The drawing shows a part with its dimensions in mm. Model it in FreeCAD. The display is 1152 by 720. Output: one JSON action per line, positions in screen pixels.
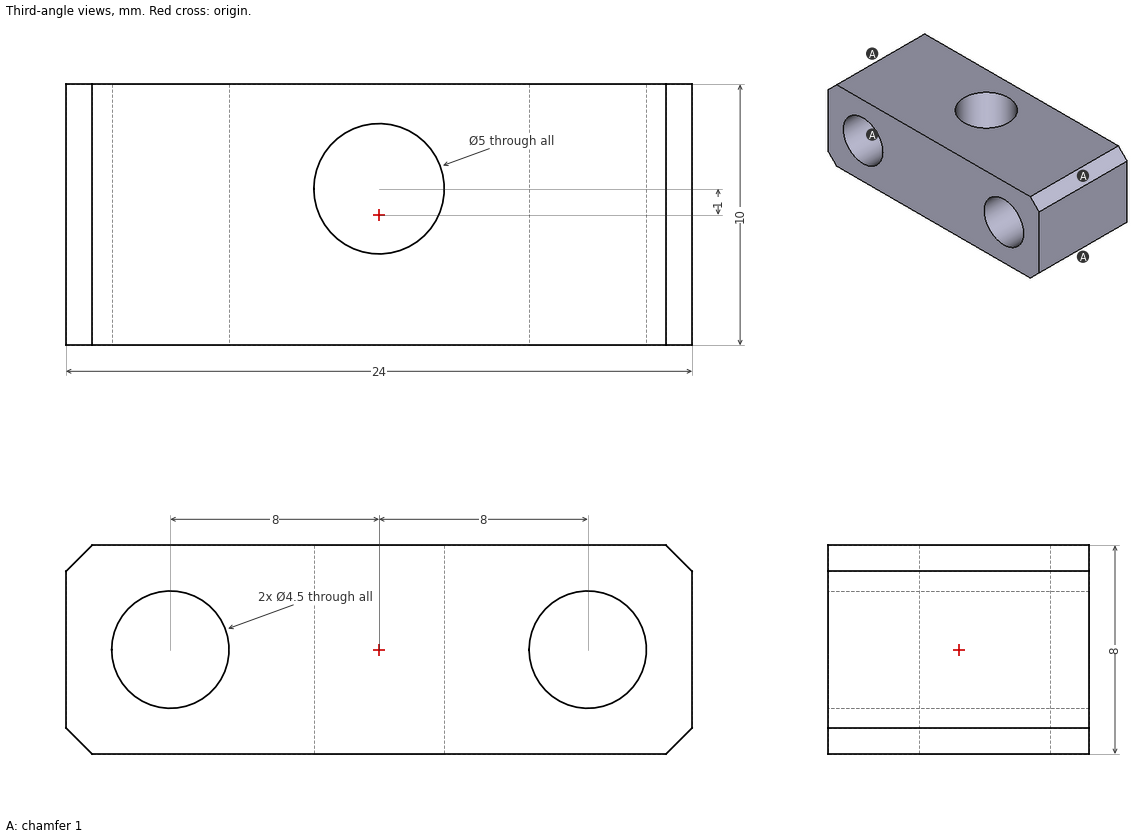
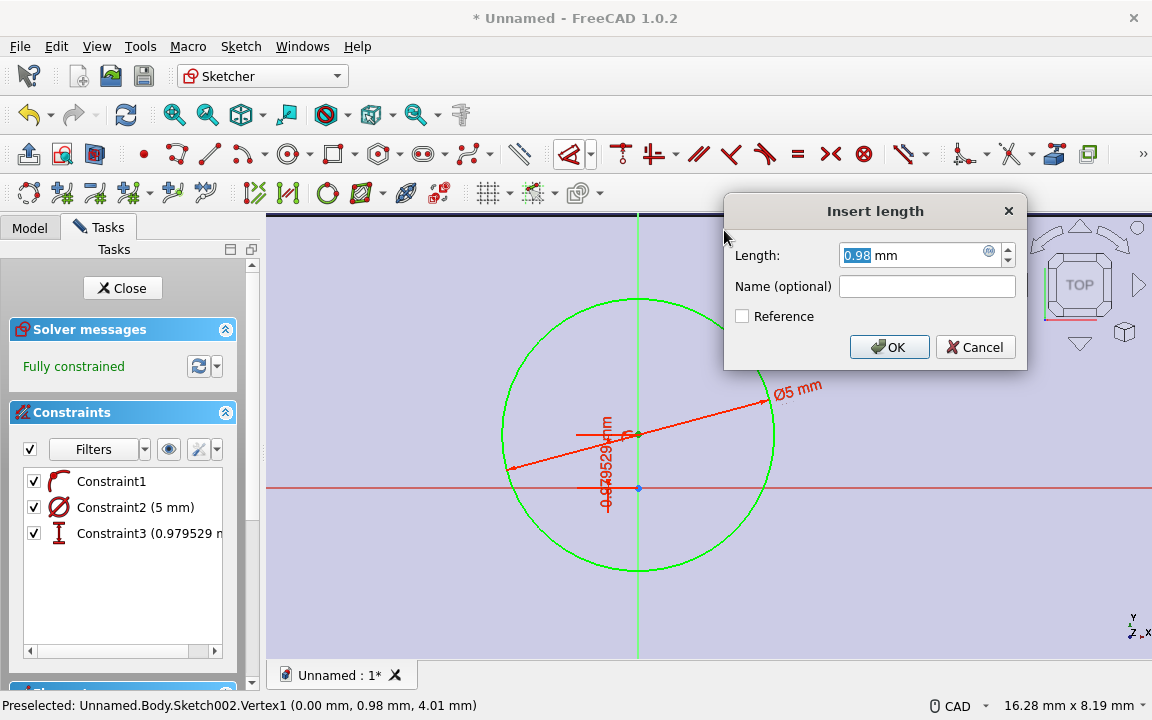
{"action": "type", "text": "1"}
{"action": "key", "text": "Return"}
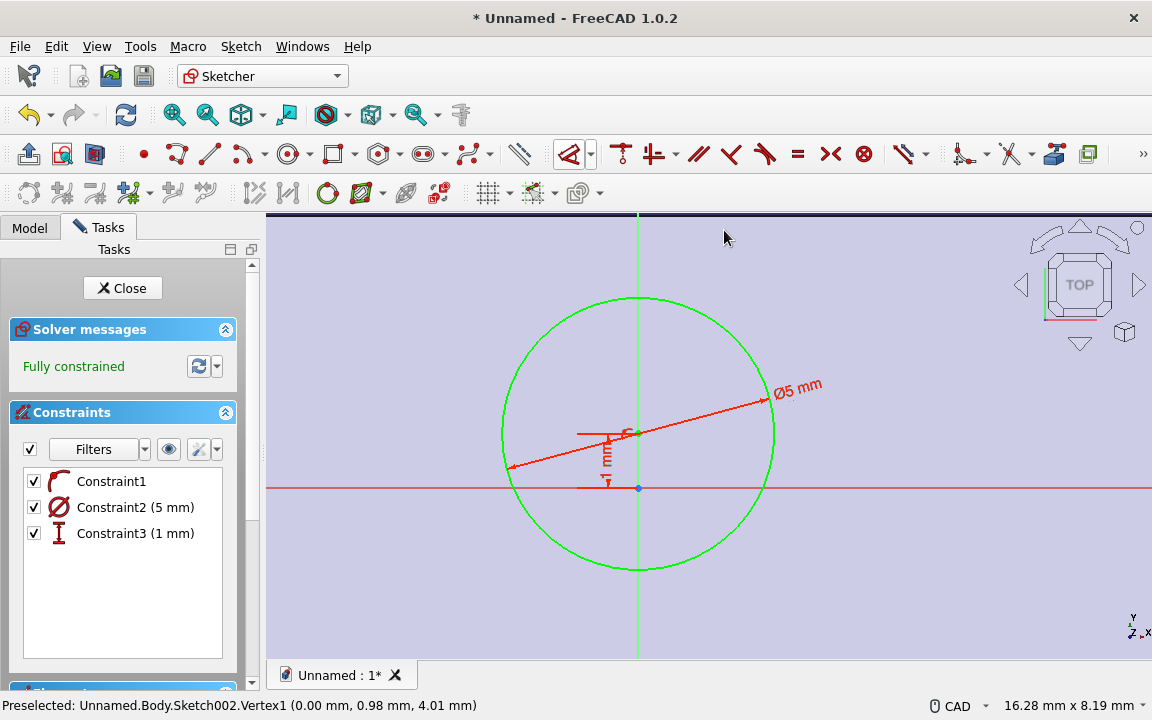
{"action": "left_click", "coordinate": [123, 288]}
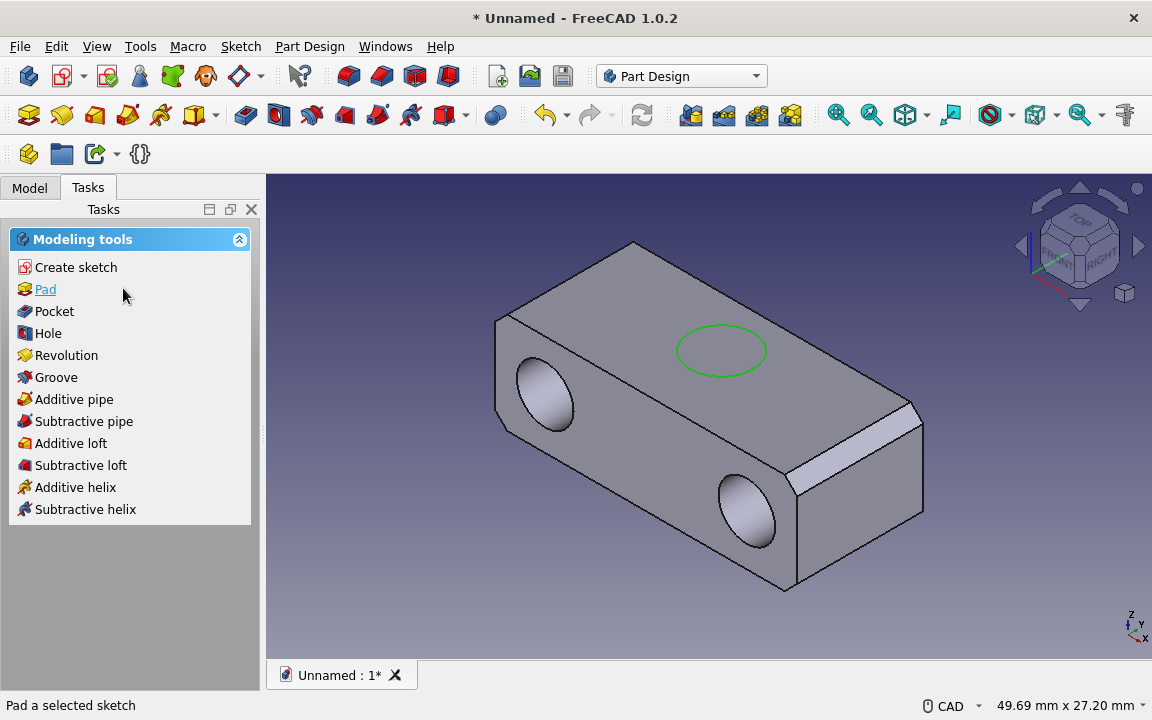
{"action": "left_click", "coordinate": [279, 116]}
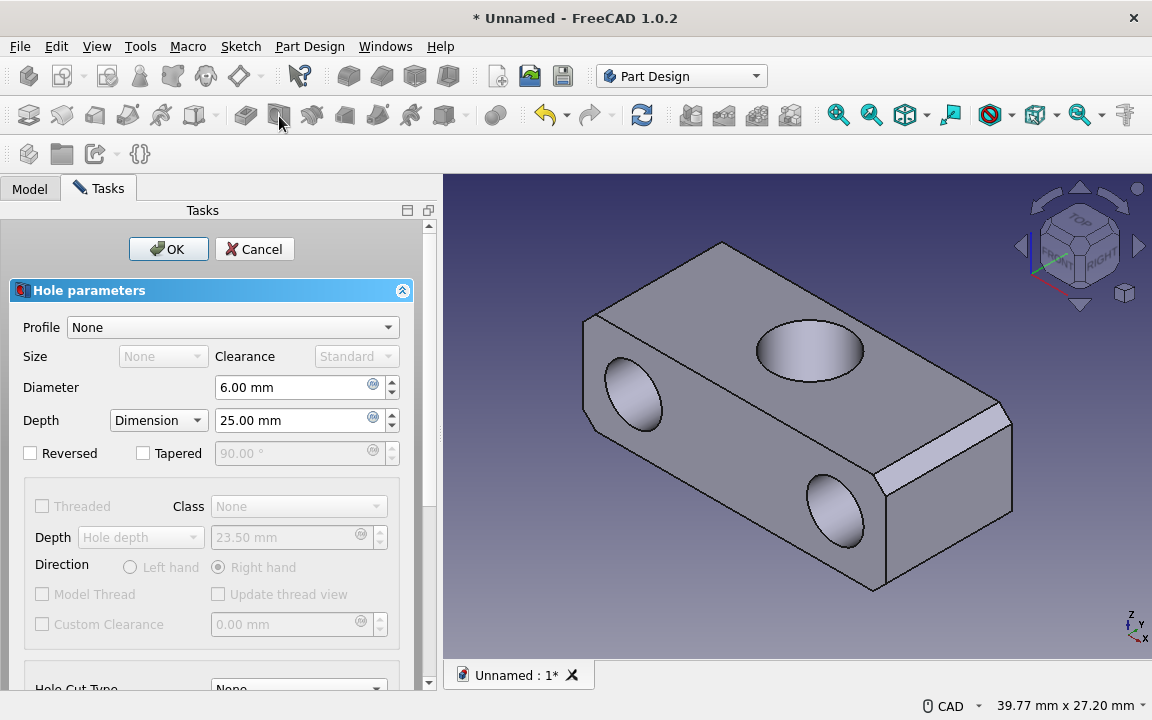
{"action": "triple_click", "coordinate": [300, 388]}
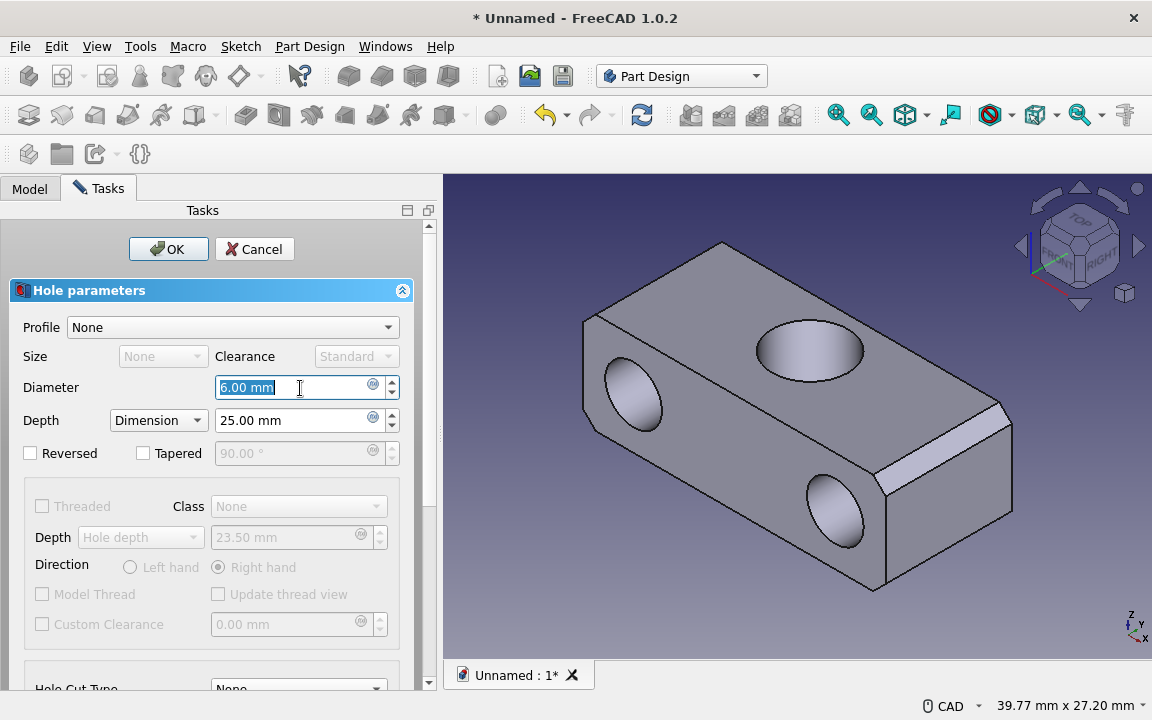
{"action": "type", "text": "5"}
{"action": "key", "text": "Tab"}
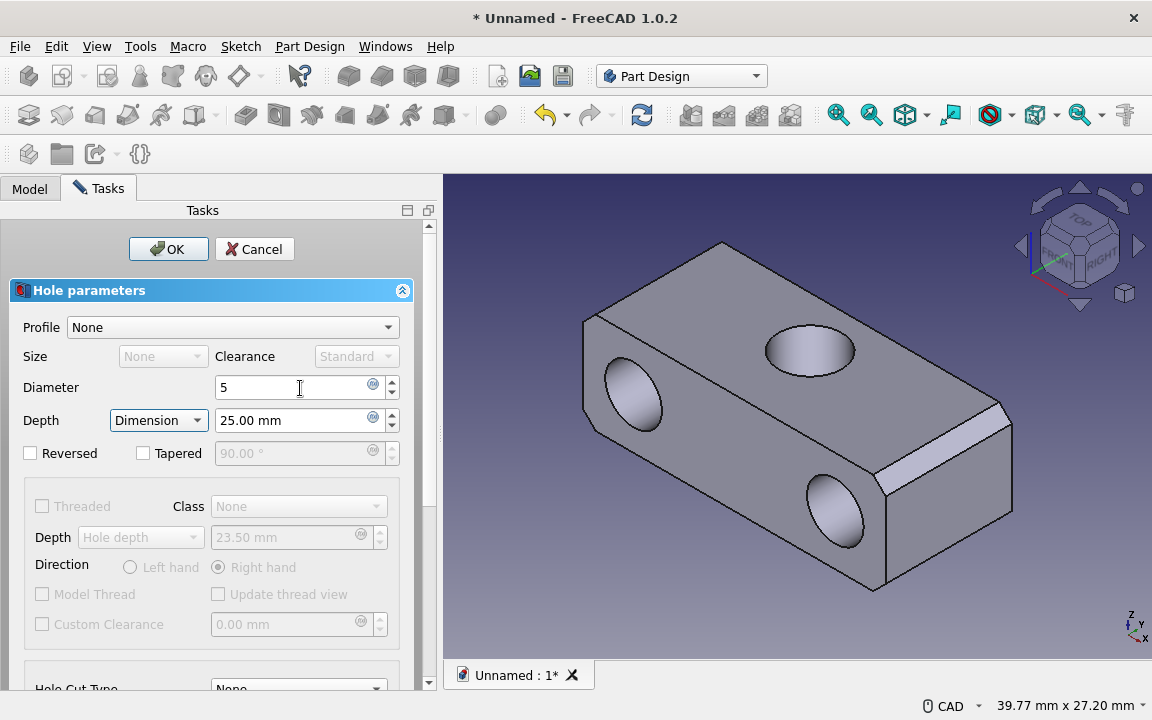
{"action": "left_click", "coordinate": [160, 420]}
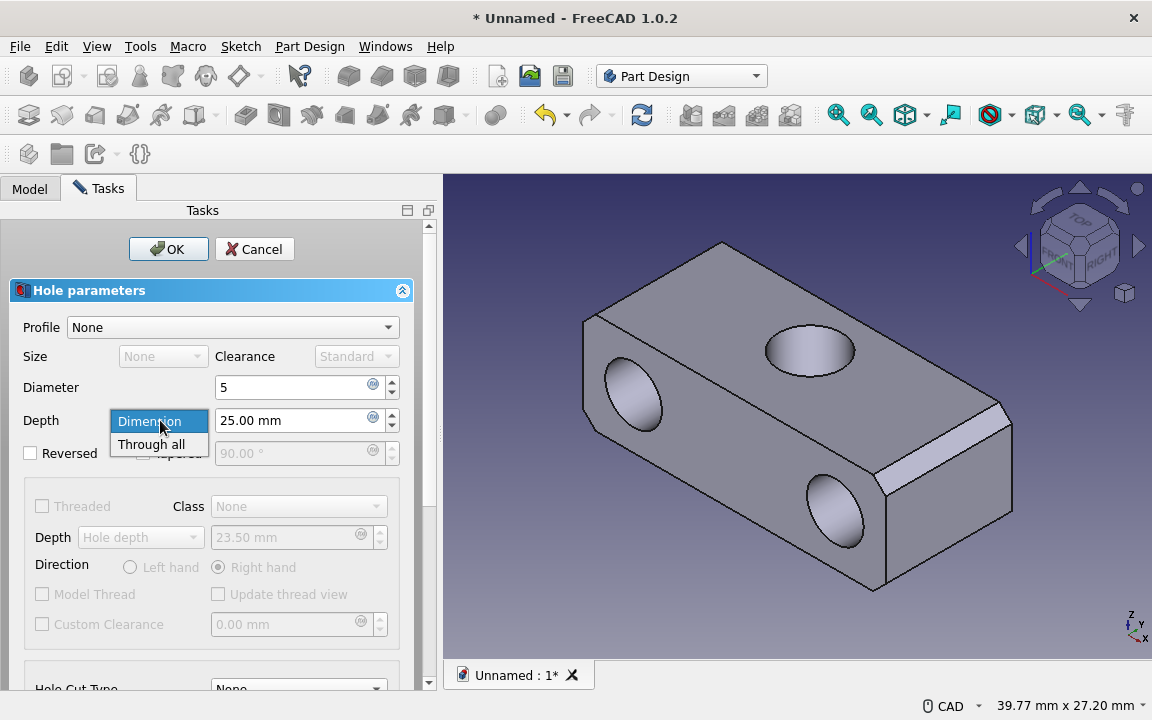
{"action": "left_click", "coordinate": [158, 444]}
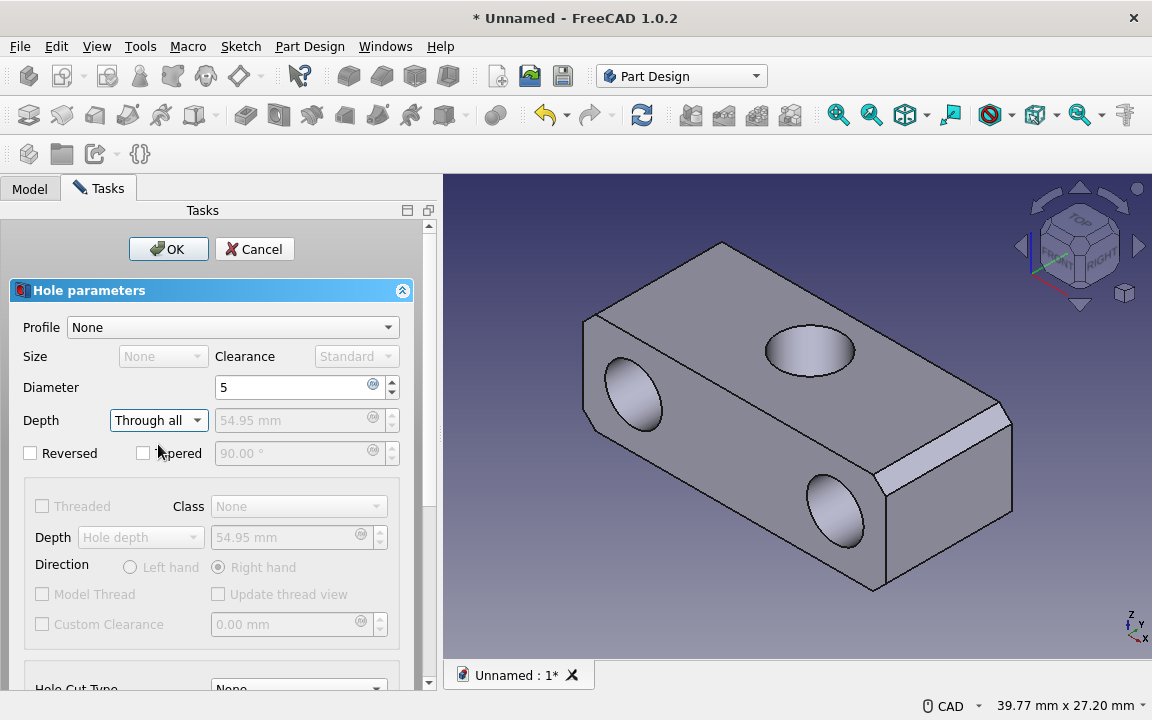
{"action": "left_click", "coordinate": [169, 249]}